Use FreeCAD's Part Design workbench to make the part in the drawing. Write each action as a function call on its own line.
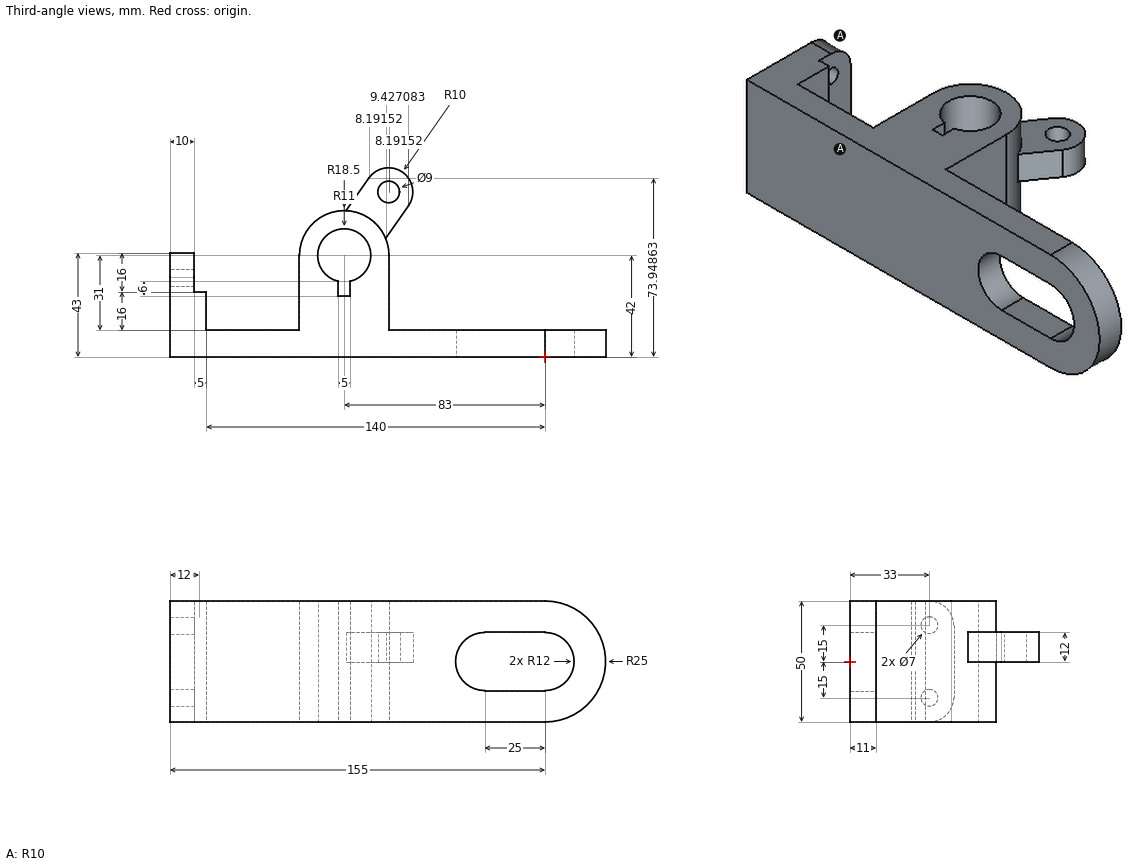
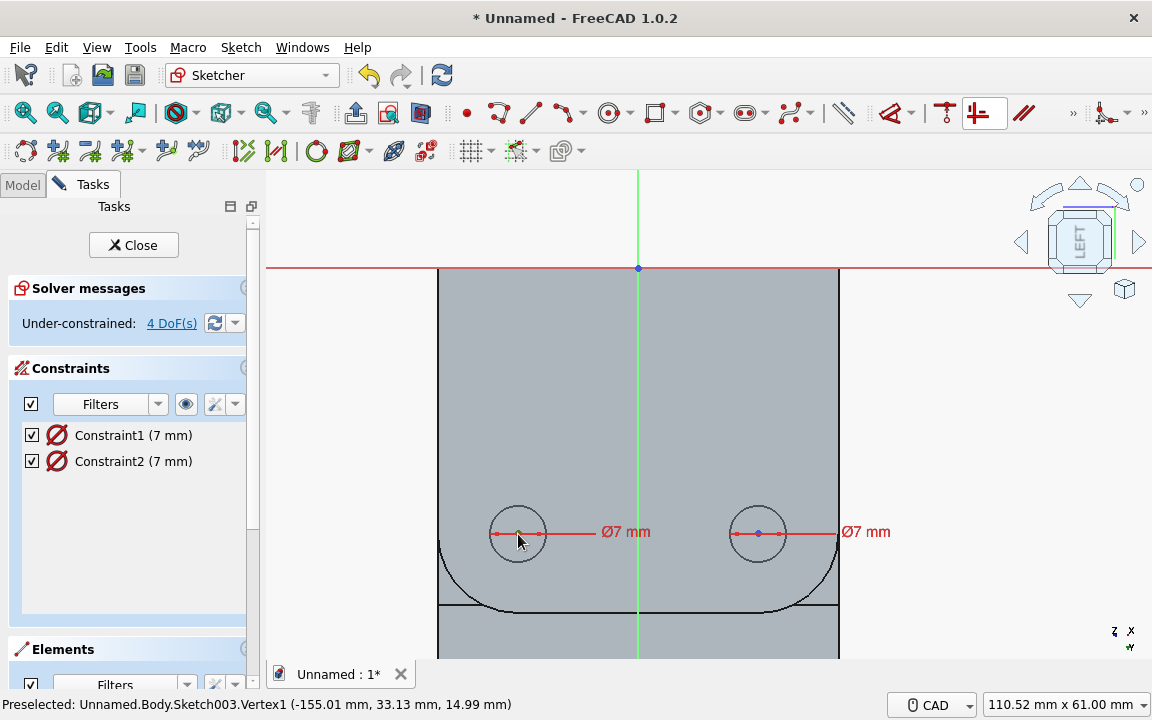
click(758, 534)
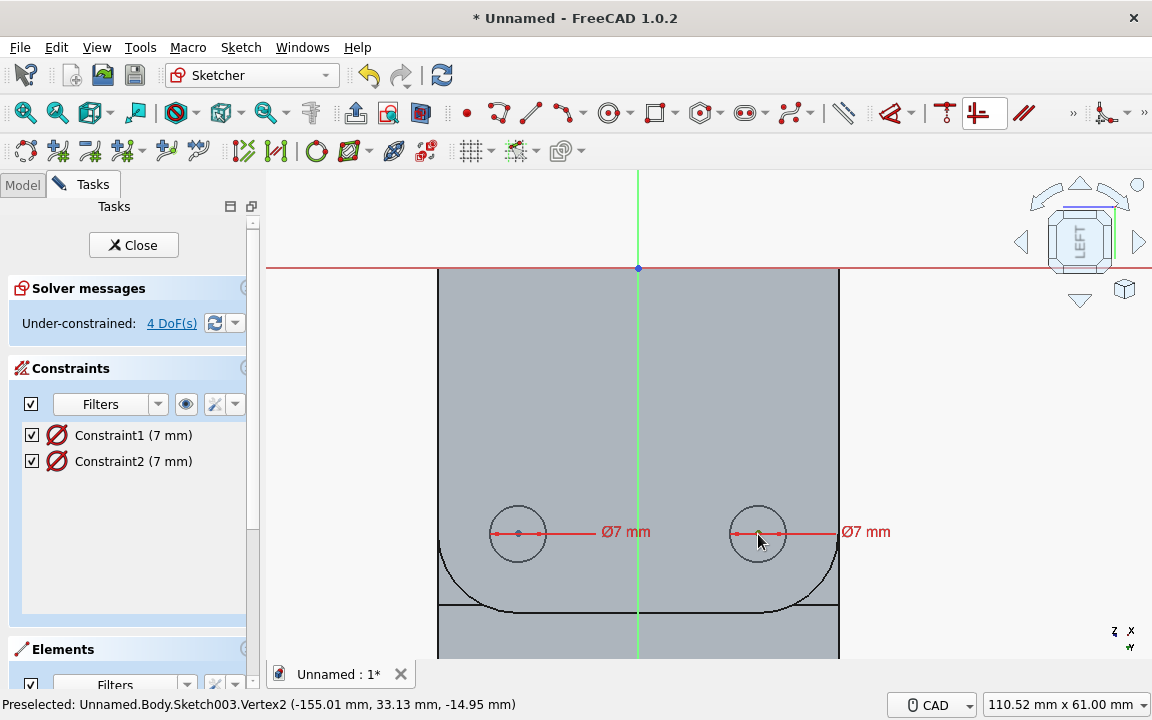
click(1002, 114)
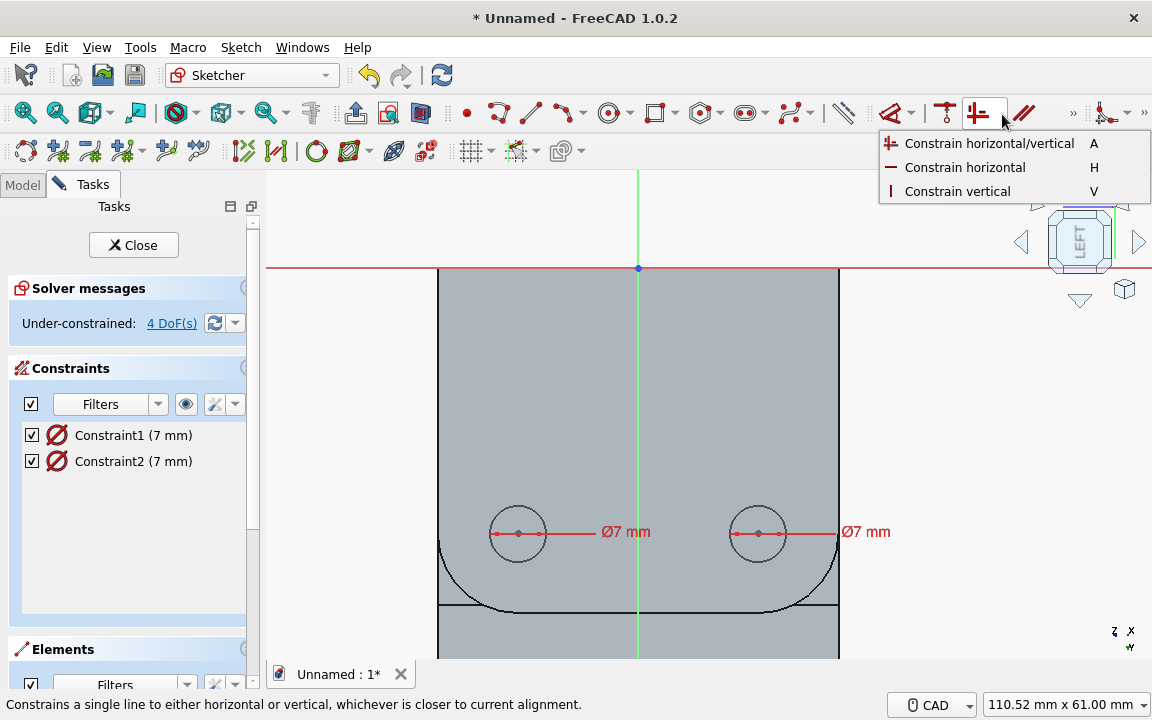
click(1015, 167)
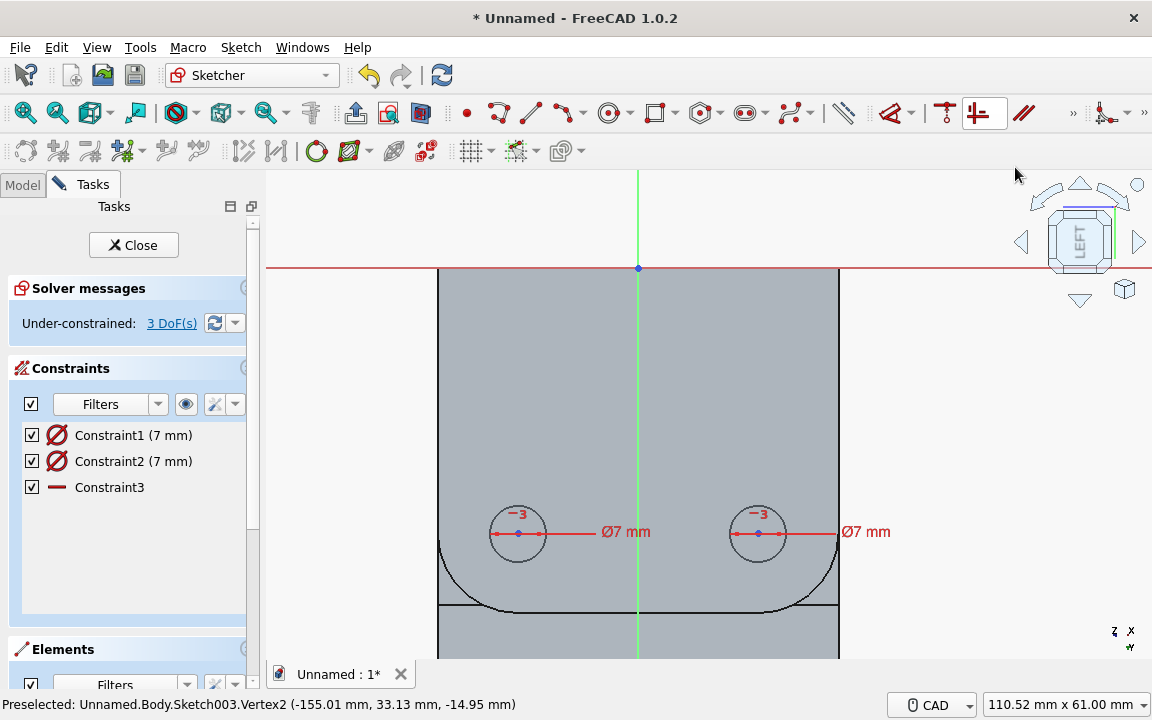
key(d)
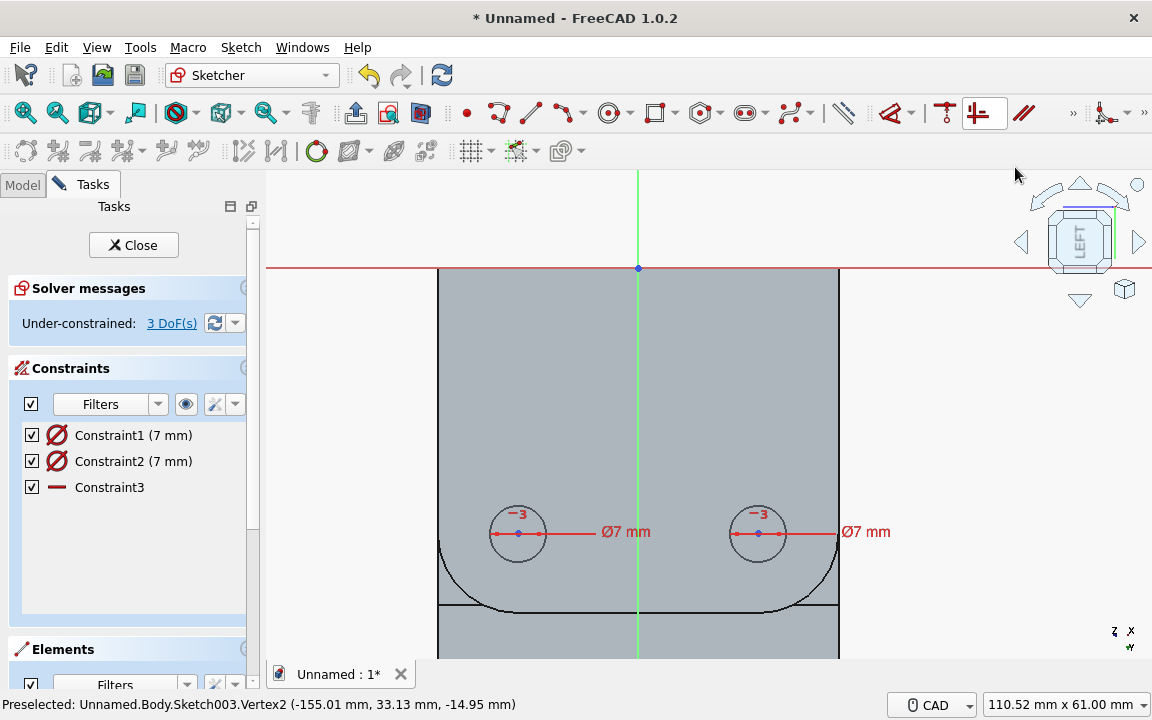
click(518, 534)
click(578, 234)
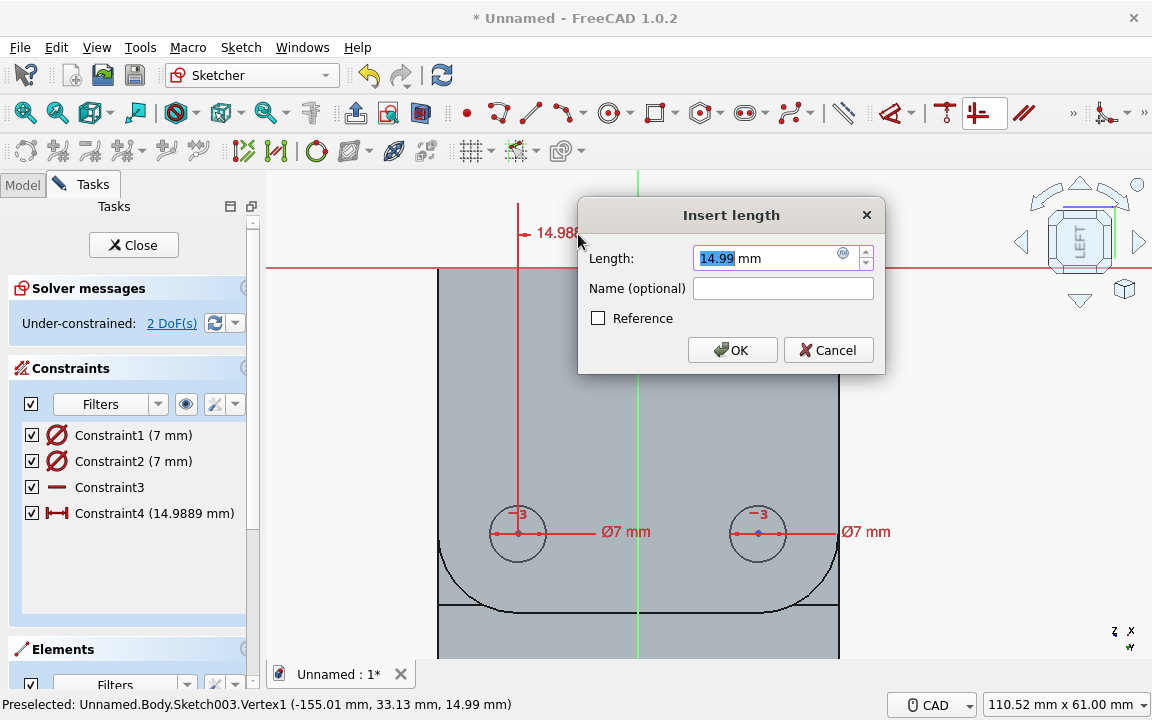
text(15)
key(Return)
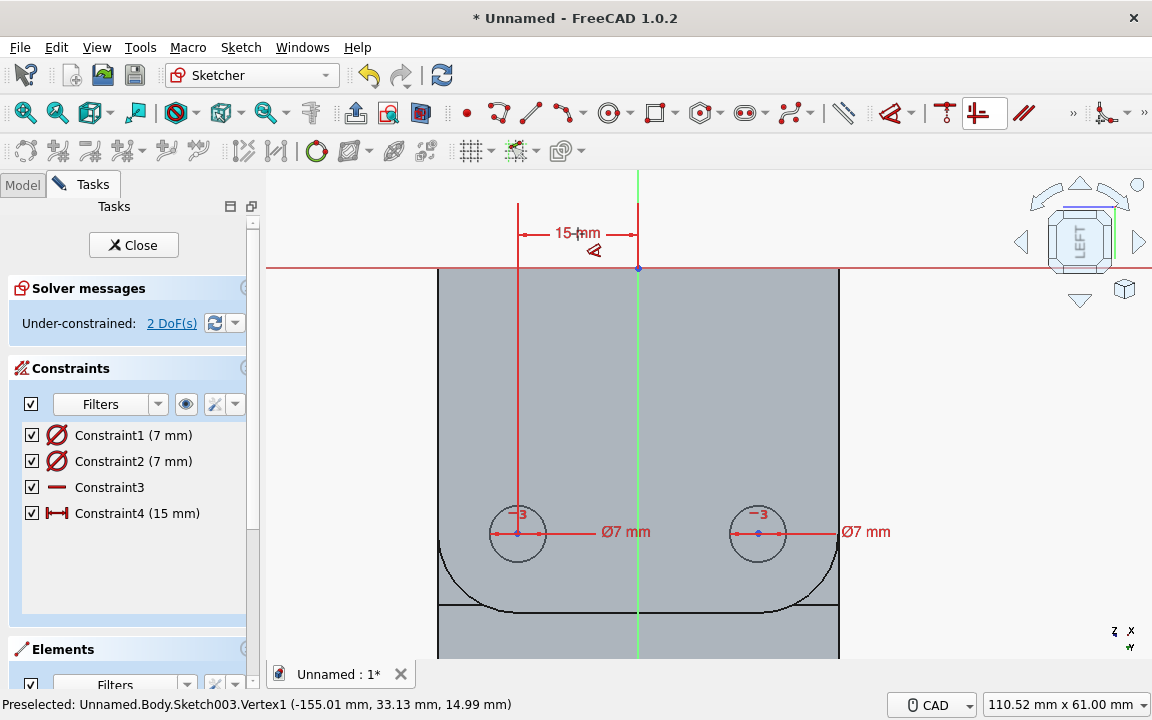
click(518, 534)
click(484, 401)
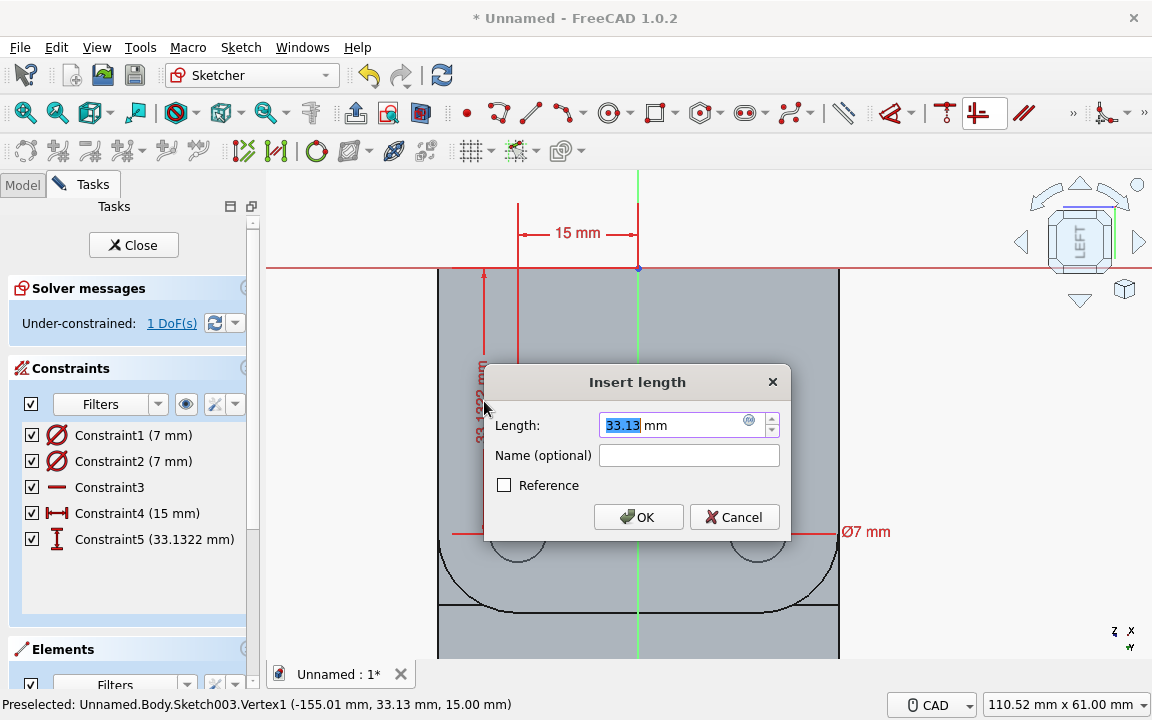
text(33)
key(Return)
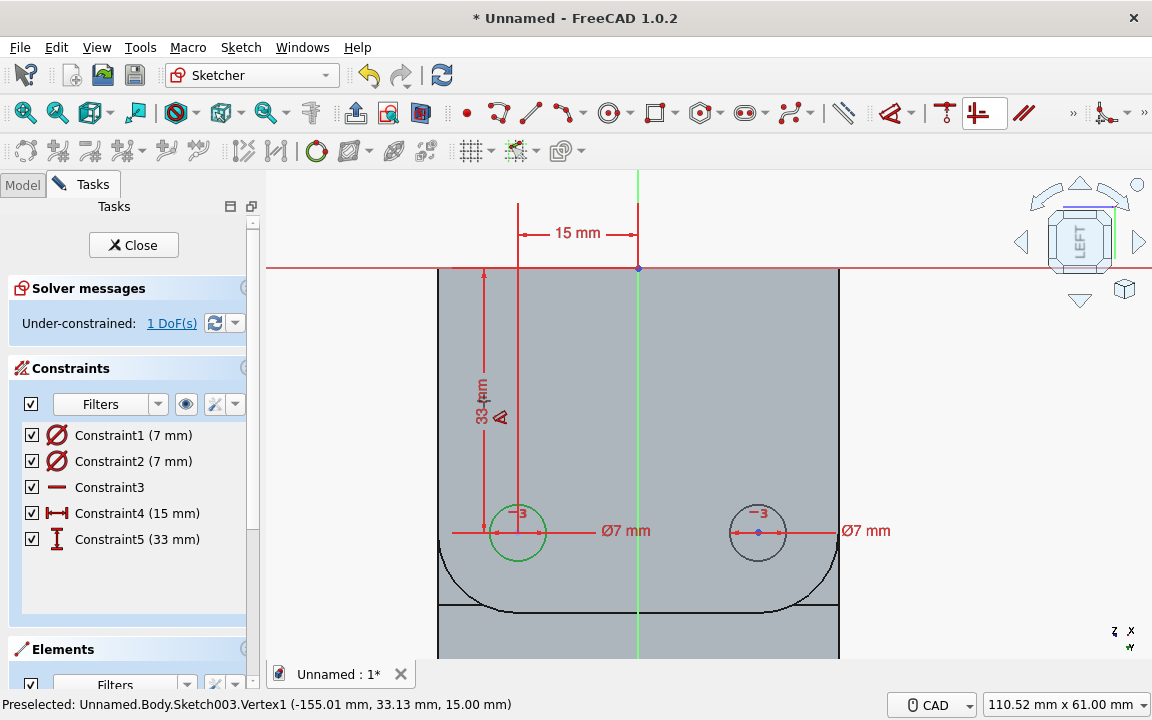
click(758, 533)
click(698, 234)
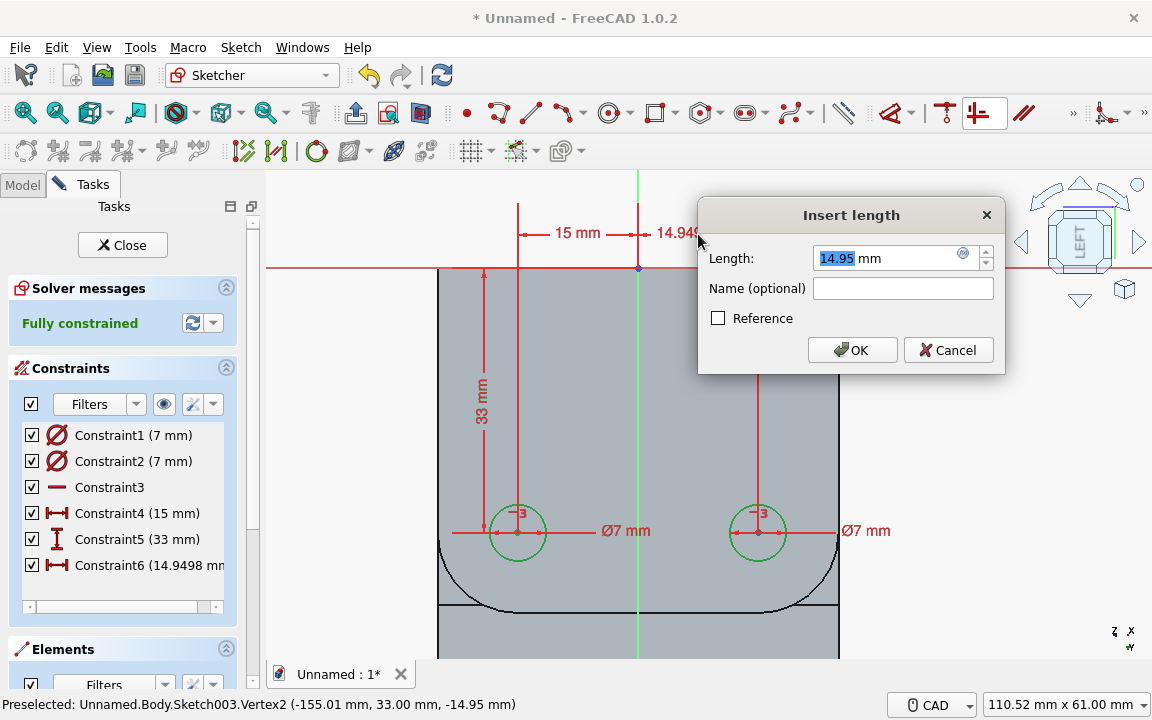
text(15)
key(Return)
key(Escape)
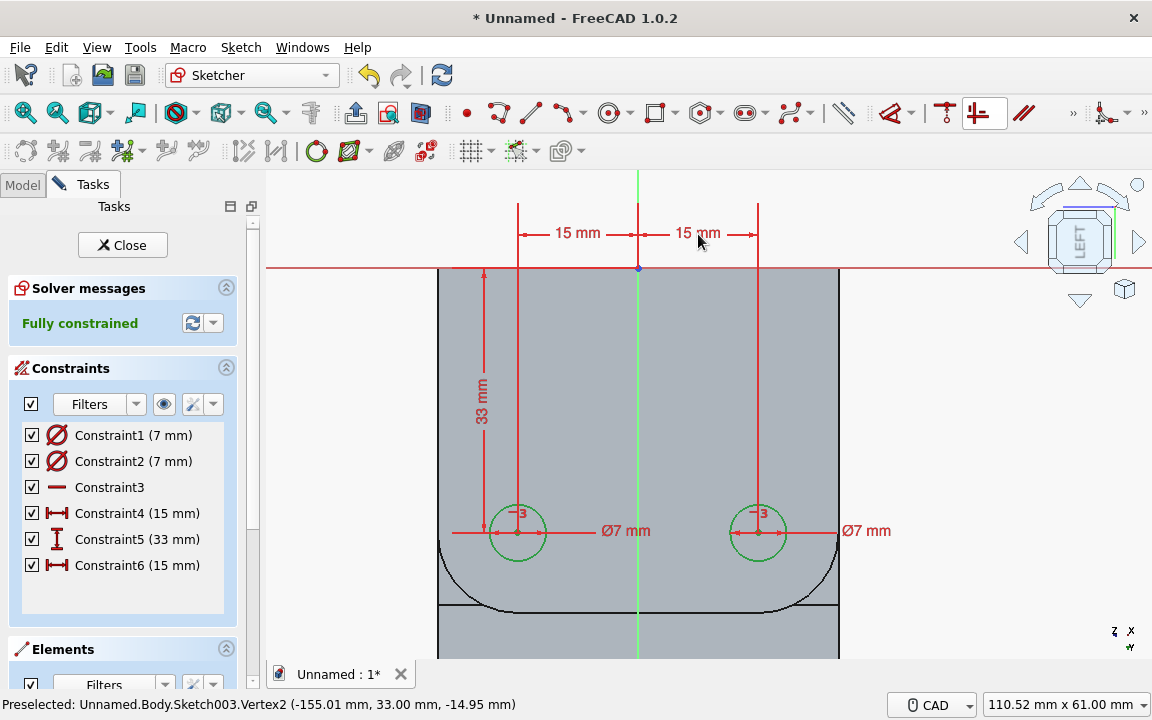
click(123, 245)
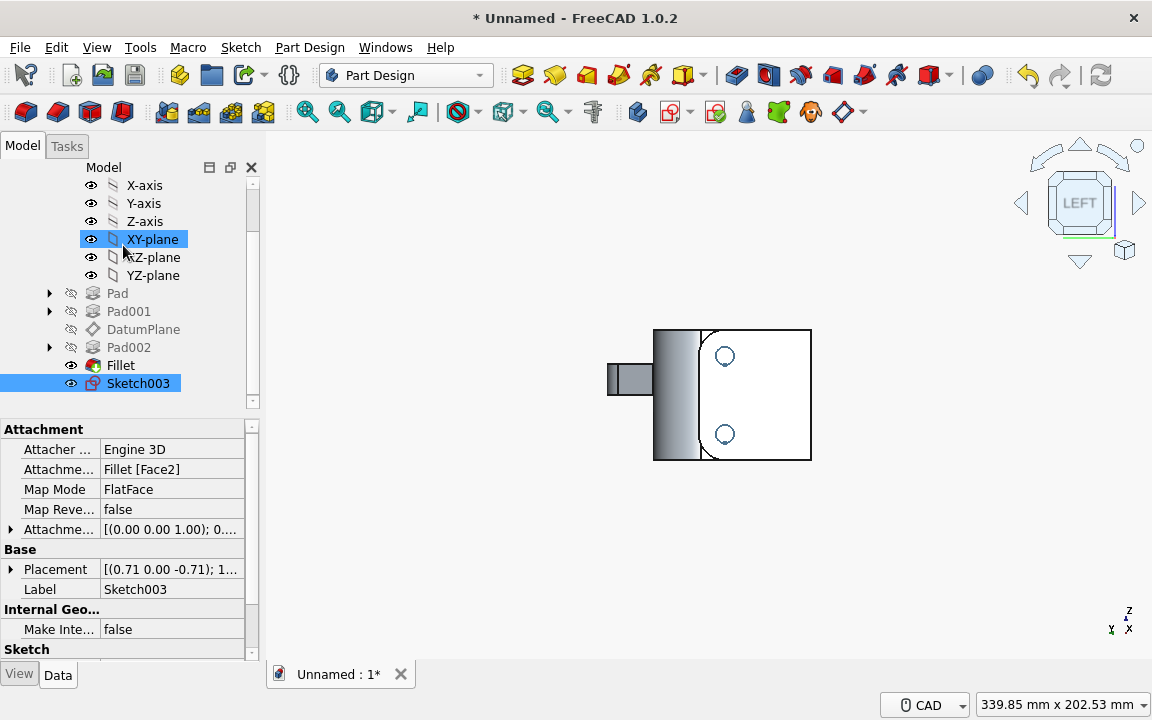
click(738, 76)